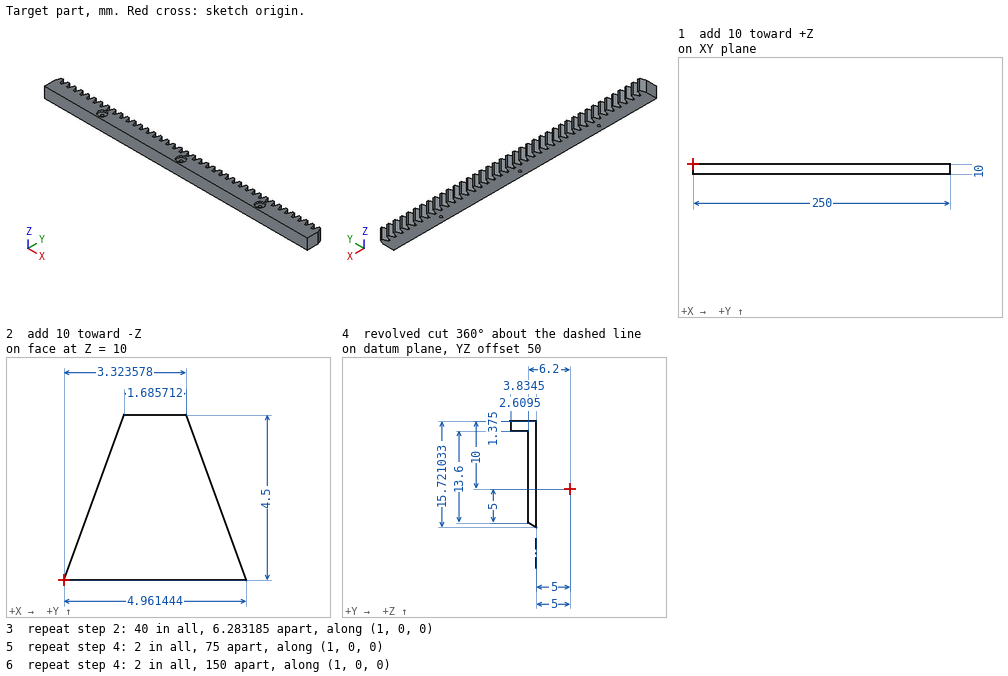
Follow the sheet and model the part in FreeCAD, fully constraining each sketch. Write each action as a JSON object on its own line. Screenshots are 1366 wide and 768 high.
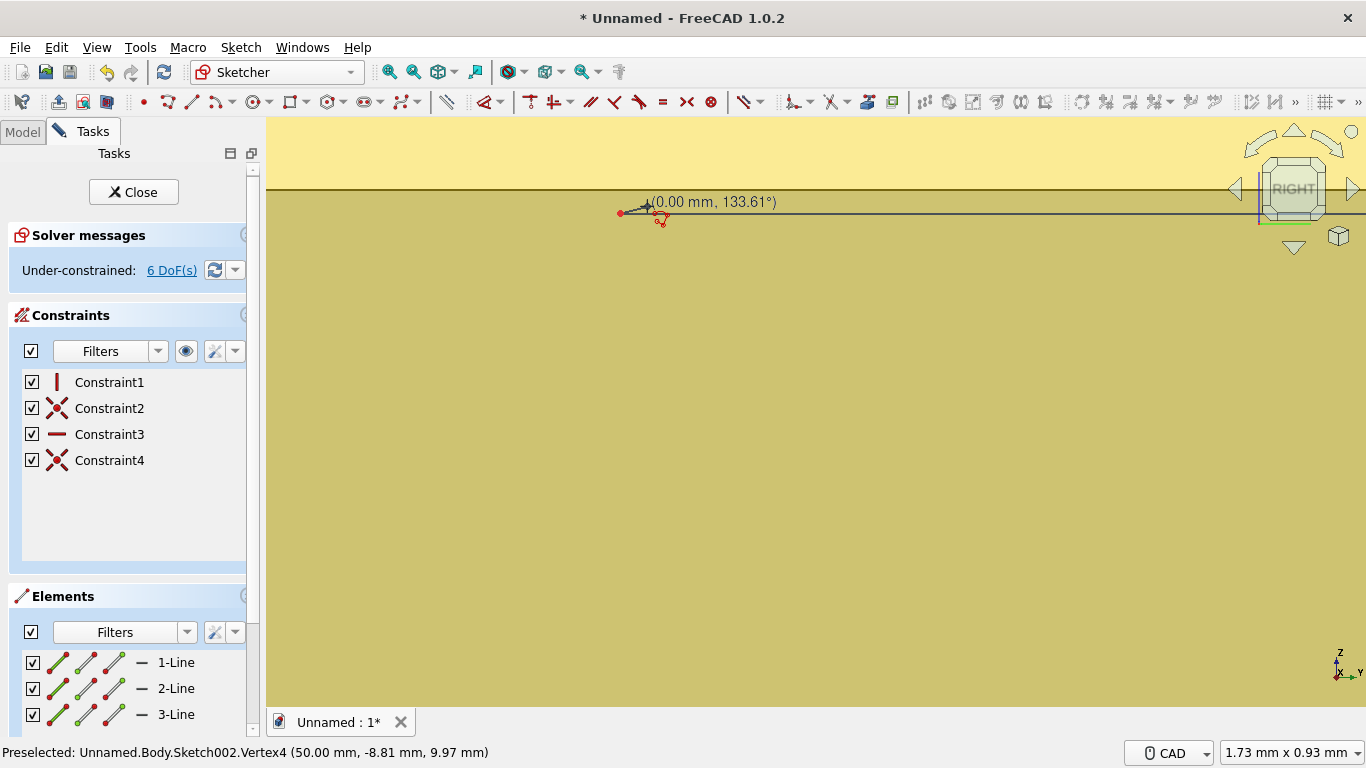
{"action": "scroll", "coordinate": [654, 178], "scroll_direction": "down", "scroll_amount": 17}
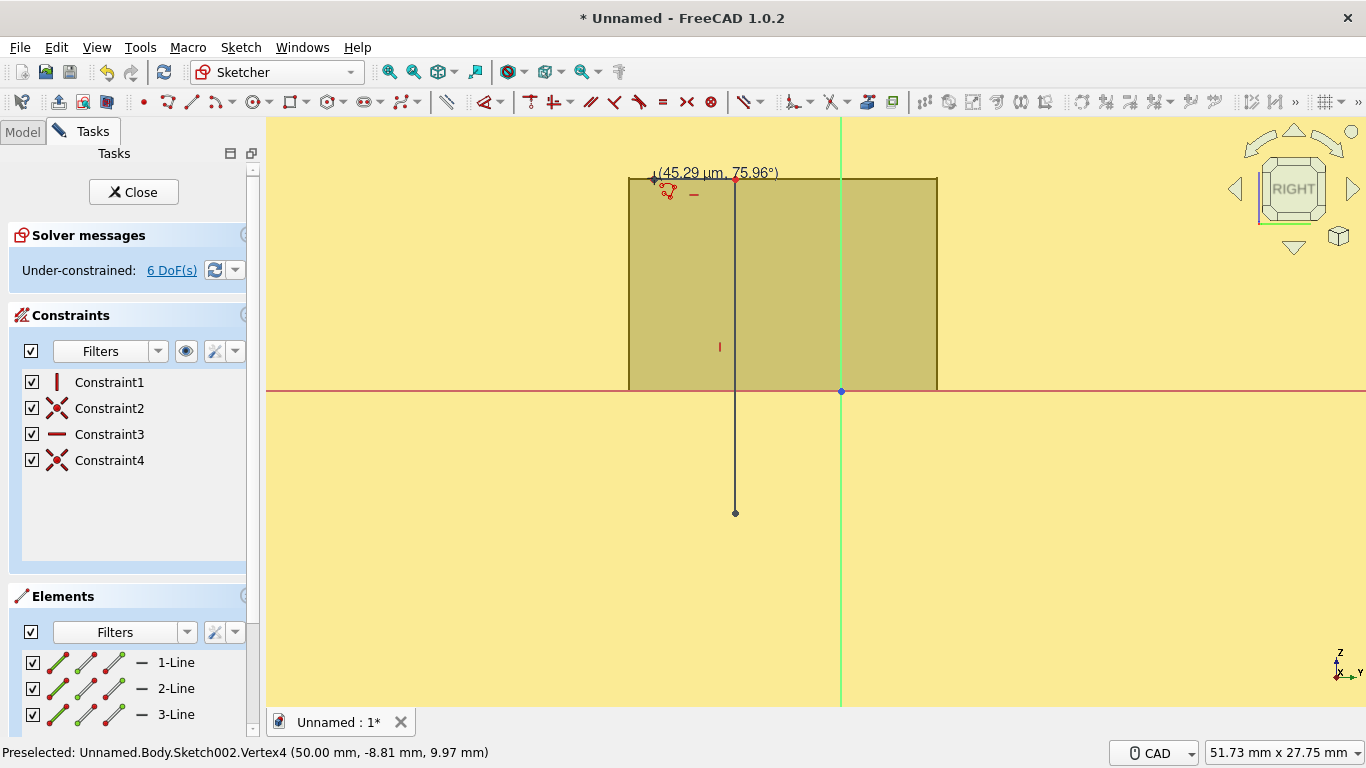
{"action": "left_click", "coordinate": [654, 208]}
{"action": "left_click", "coordinate": [710, 208]}
{"action": "left_click", "coordinate": [710, 497]}
{"action": "left_click", "coordinate": [735, 514]}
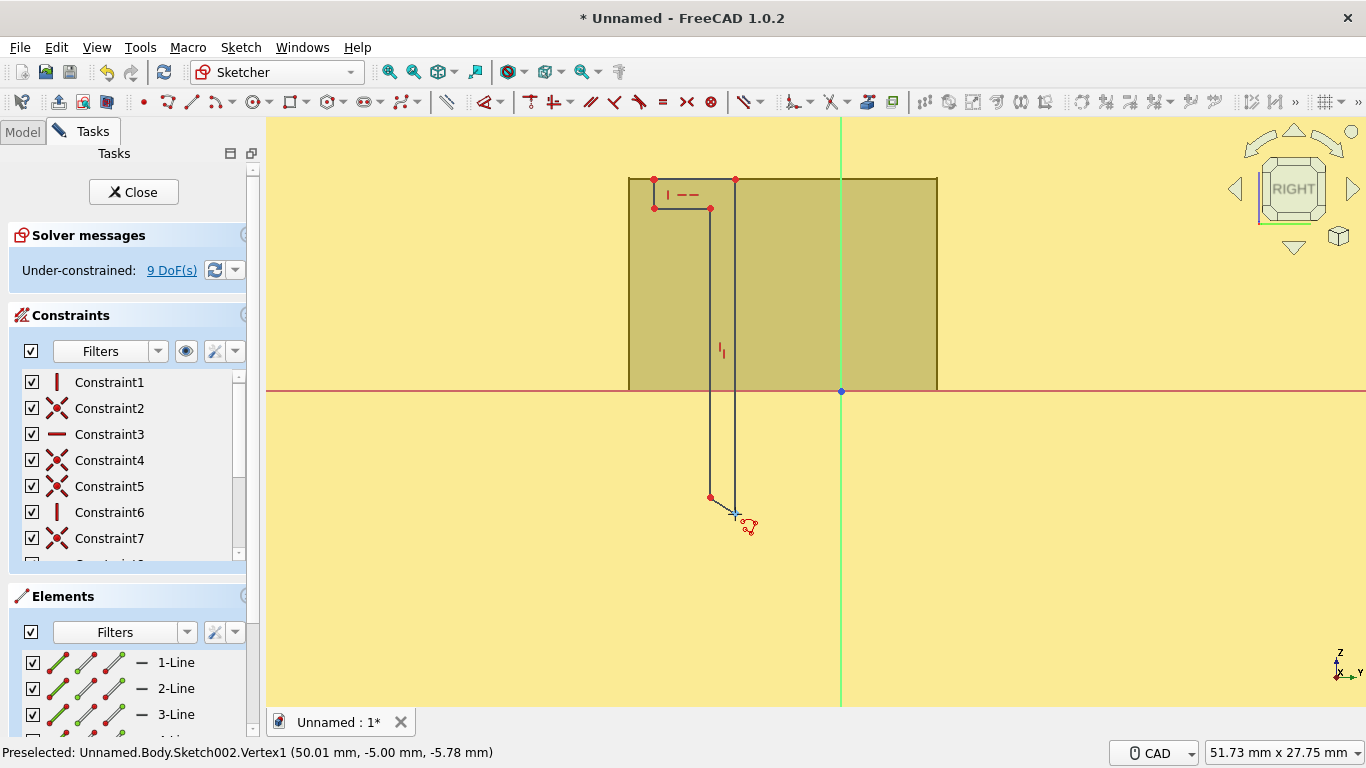
{"action": "key", "text": "g l"}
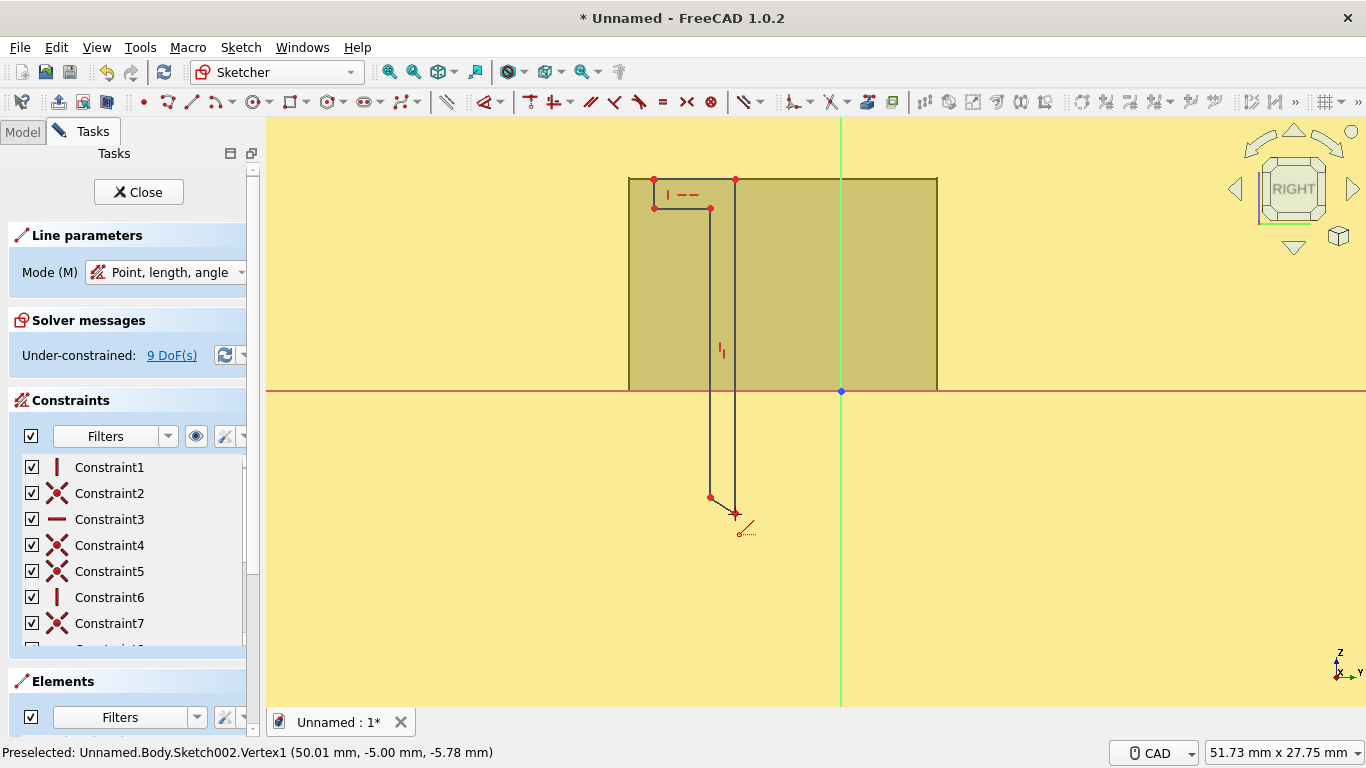
{"action": "left_click", "coordinate": [735, 546]}
{"action": "left_click", "coordinate": [735, 647]}
{"action": "key", "text": "Escape"}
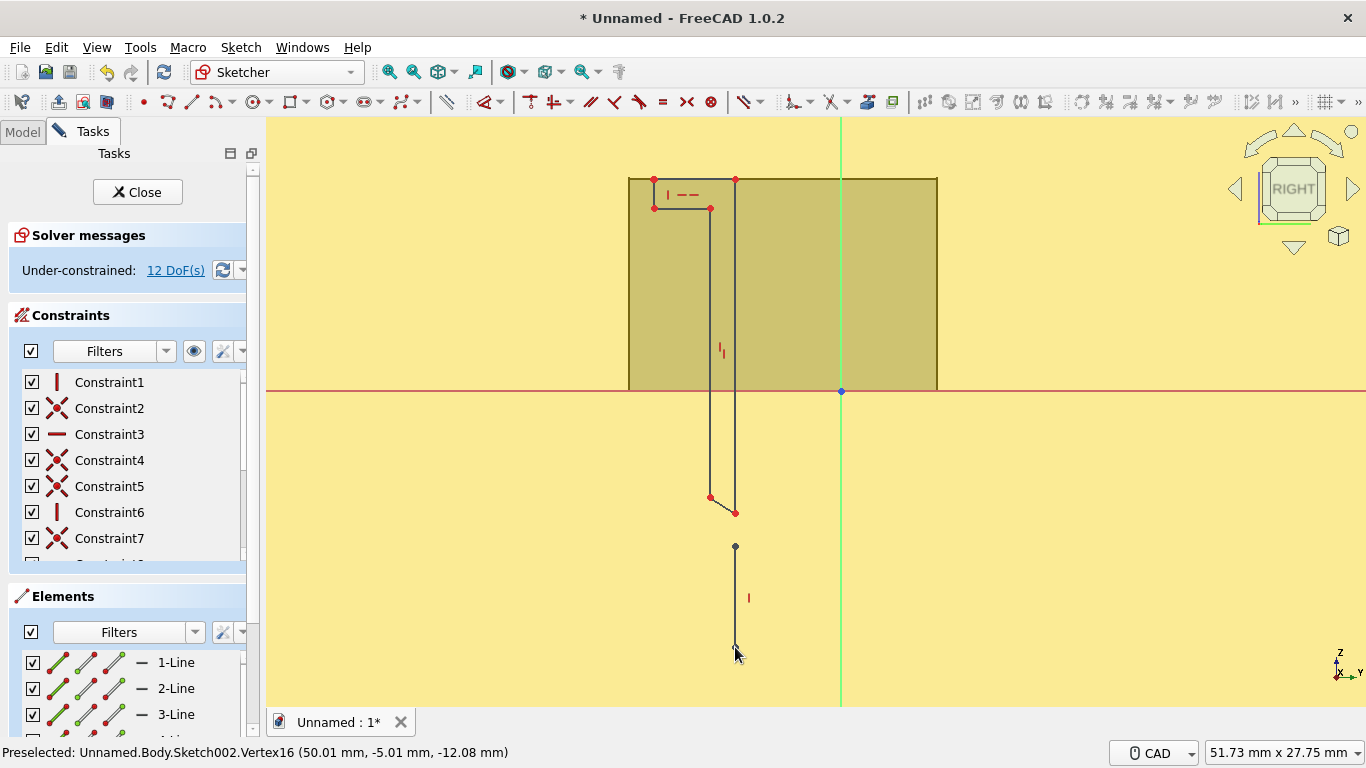
{"action": "left_click", "coordinate": [735, 577]}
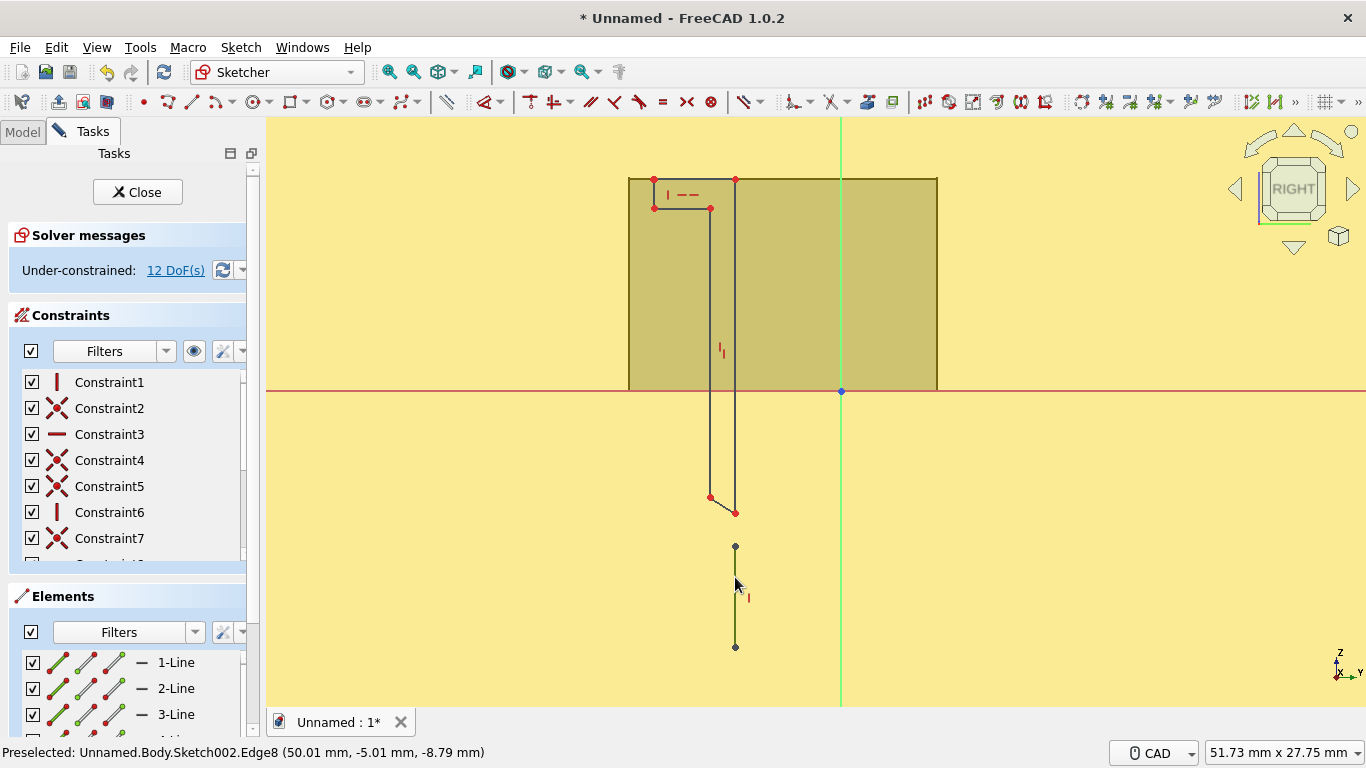
{"action": "left_click", "coordinate": [448, 102]}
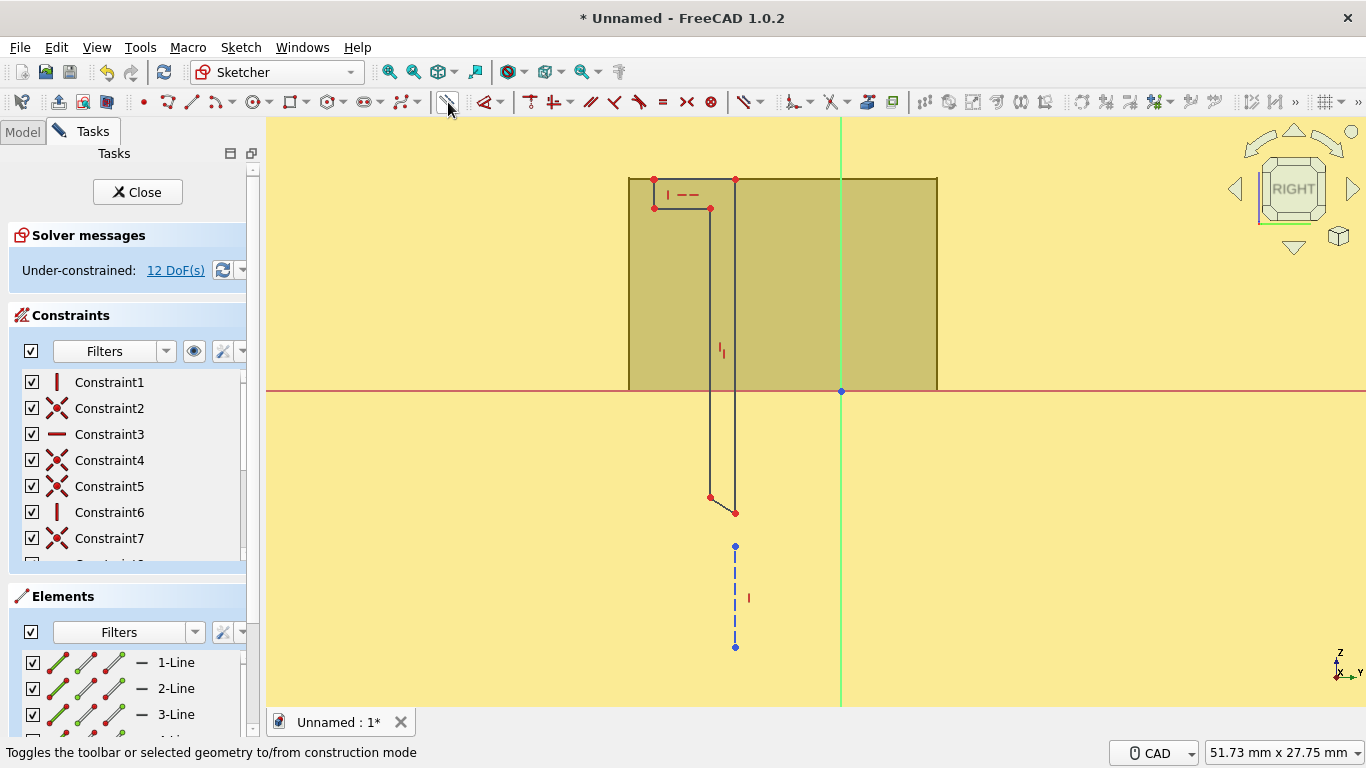
{"action": "key", "text": "d"}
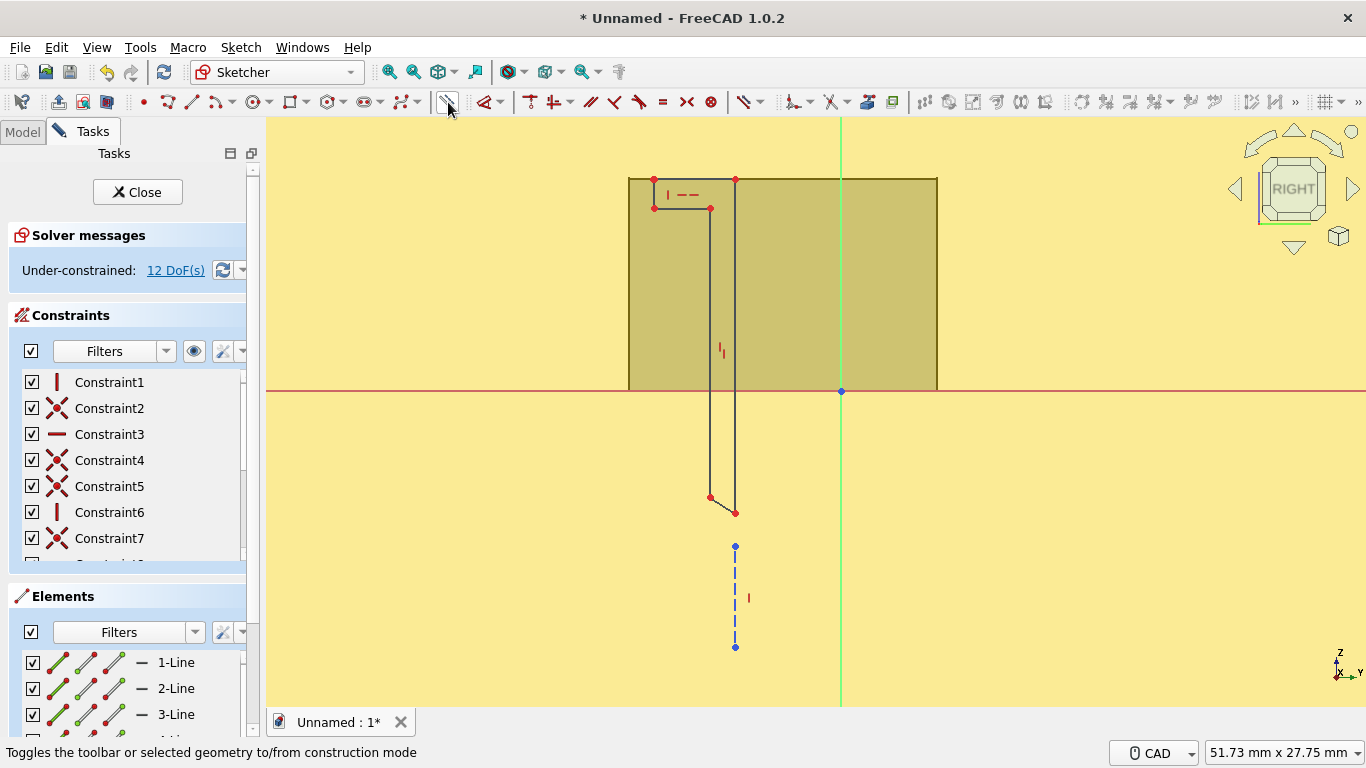
{"action": "left_click", "coordinate": [735, 514]}
{"action": "left_click", "coordinate": [788, 548]}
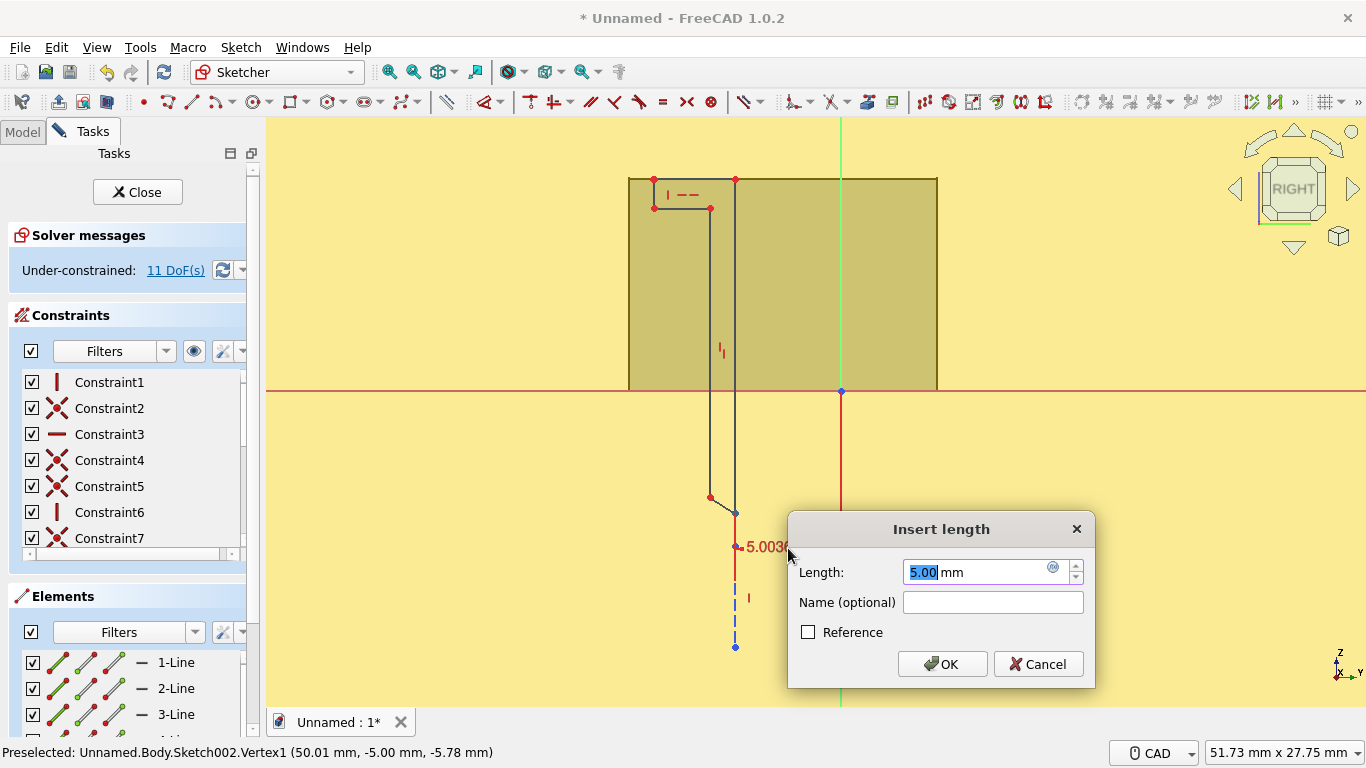
{"action": "type", "text": "5"}
{"action": "key", "text": "Return"}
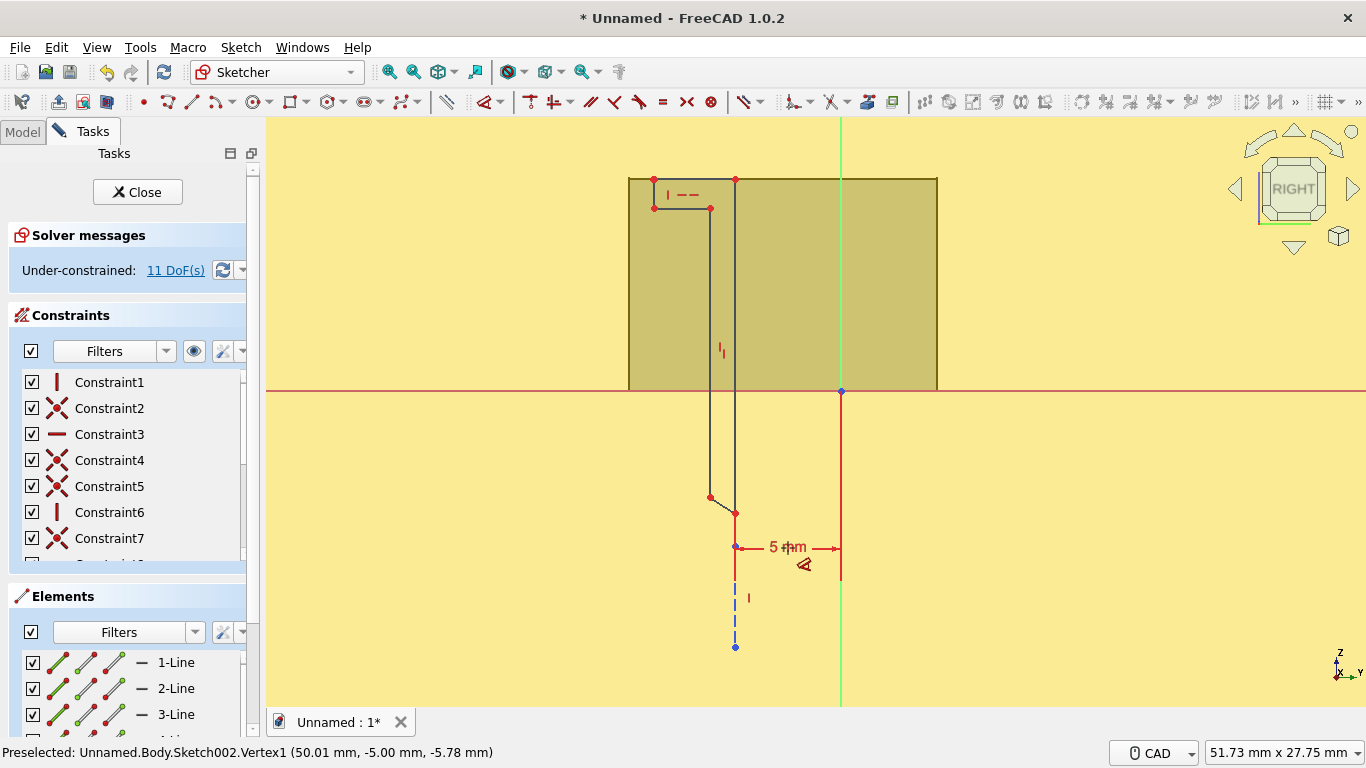
{"action": "left_click", "coordinate": [710, 498]}
{"action": "left_click", "coordinate": [875, 445]}